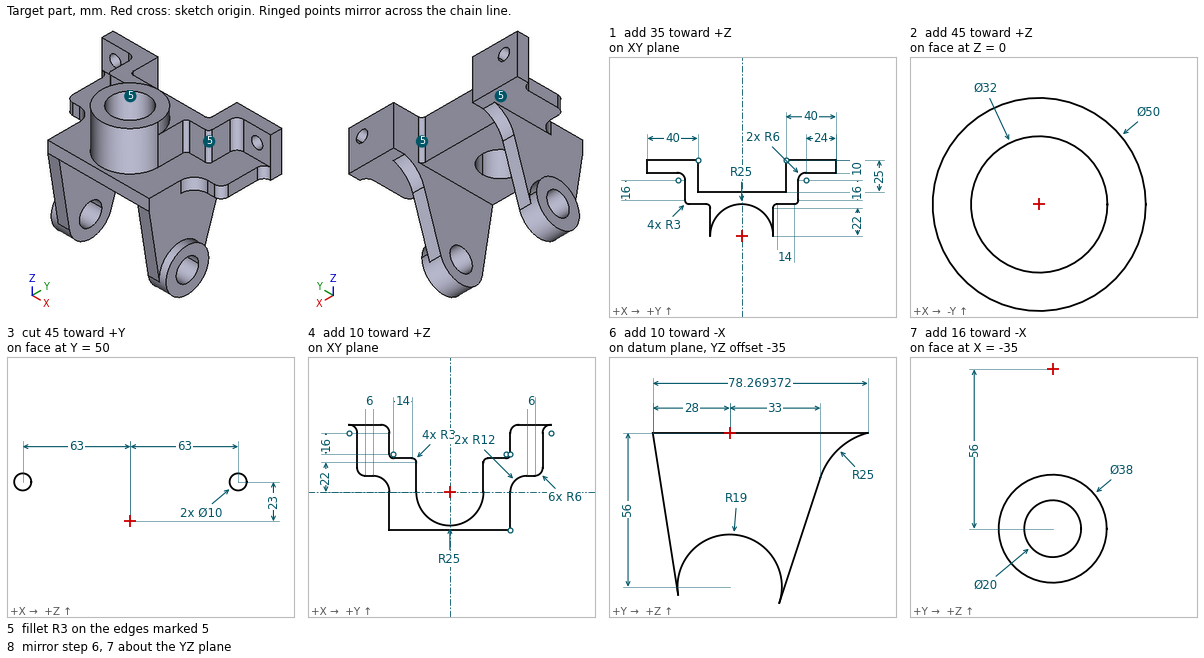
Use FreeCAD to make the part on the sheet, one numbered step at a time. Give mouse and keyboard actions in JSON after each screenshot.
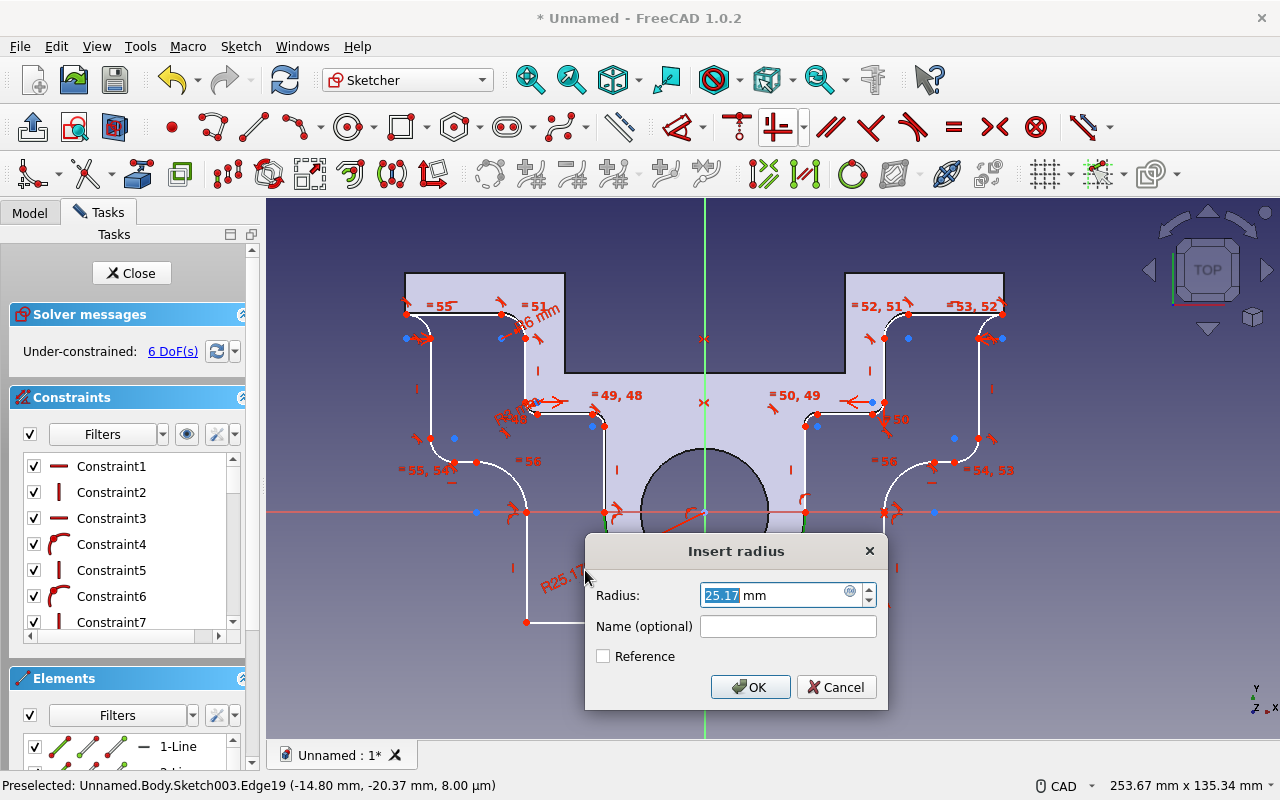
{"action": "type", "text": "25"}
{"action": "key", "text": "Return"}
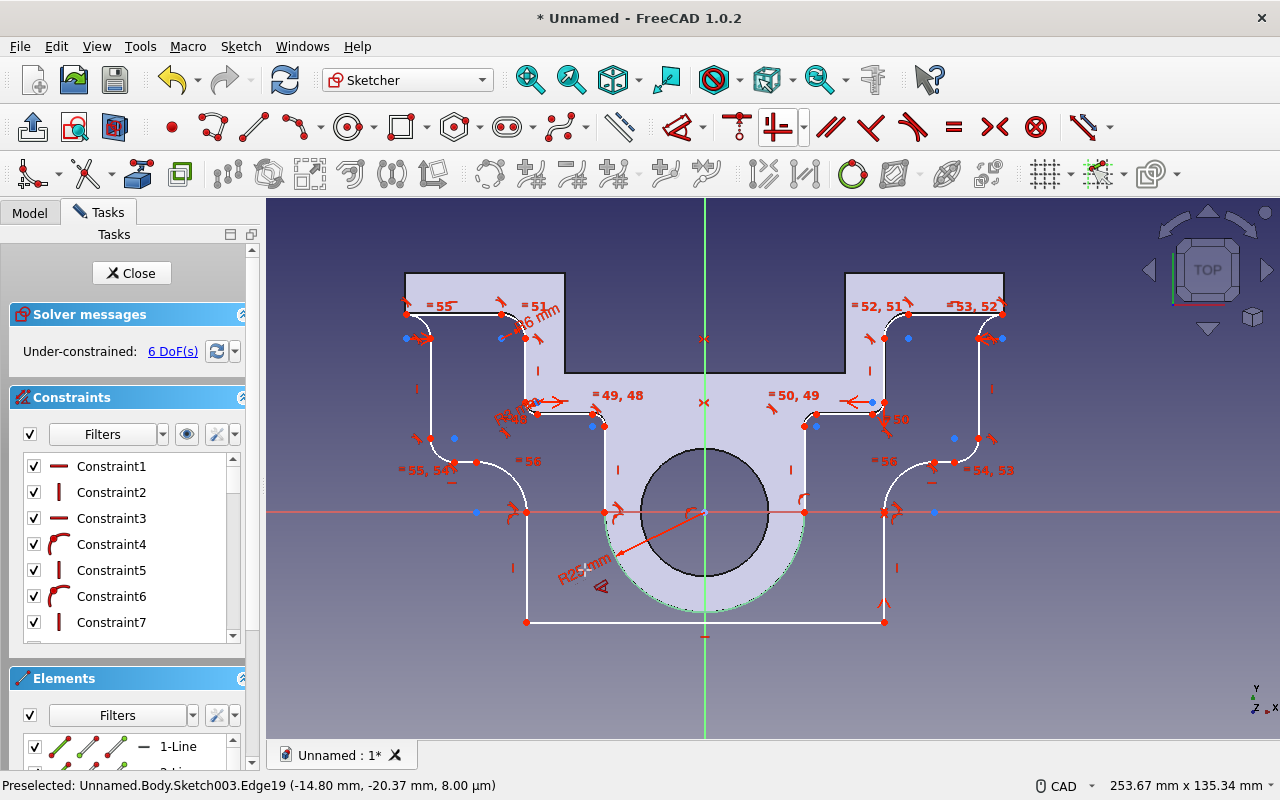
{"action": "left_click", "coordinate": [912, 468]}
{"action": "left_click", "coordinate": [898, 439]}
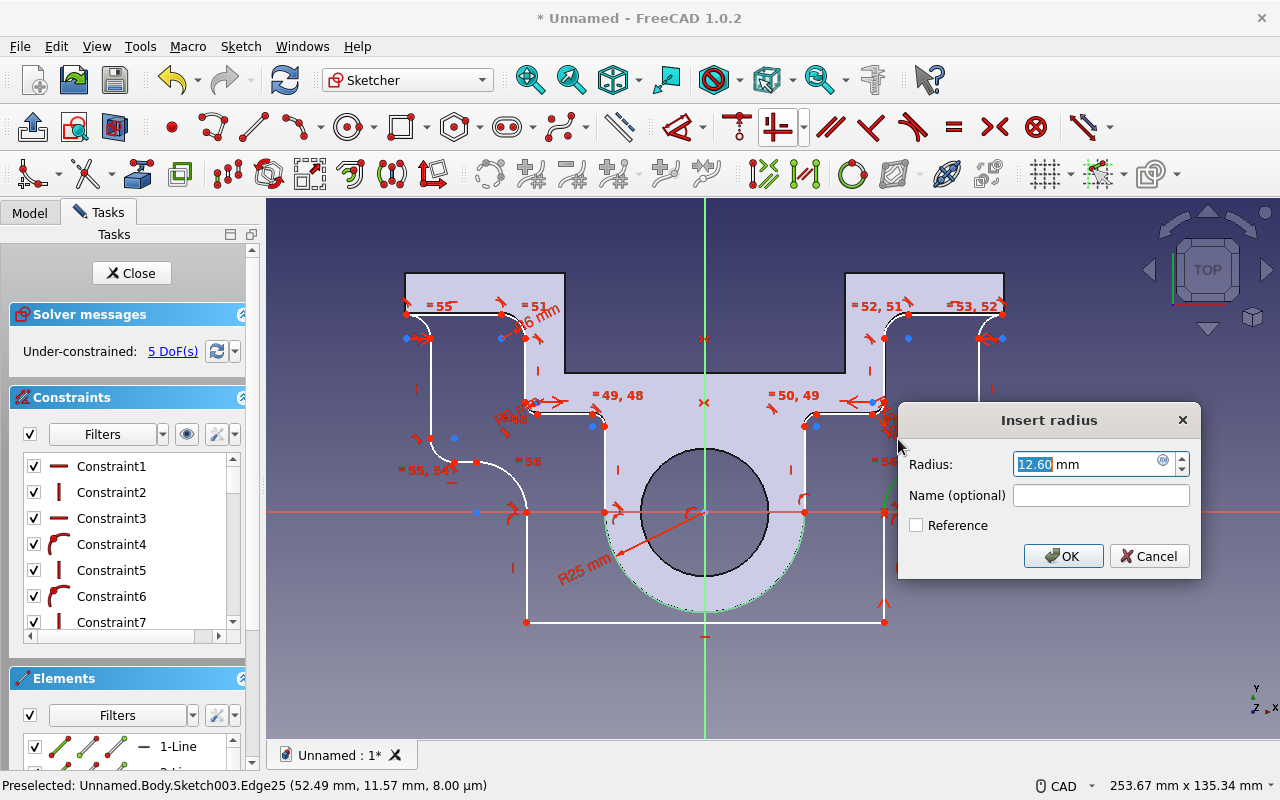
{"action": "type", "text": "12"}
{"action": "key", "text": "Return"}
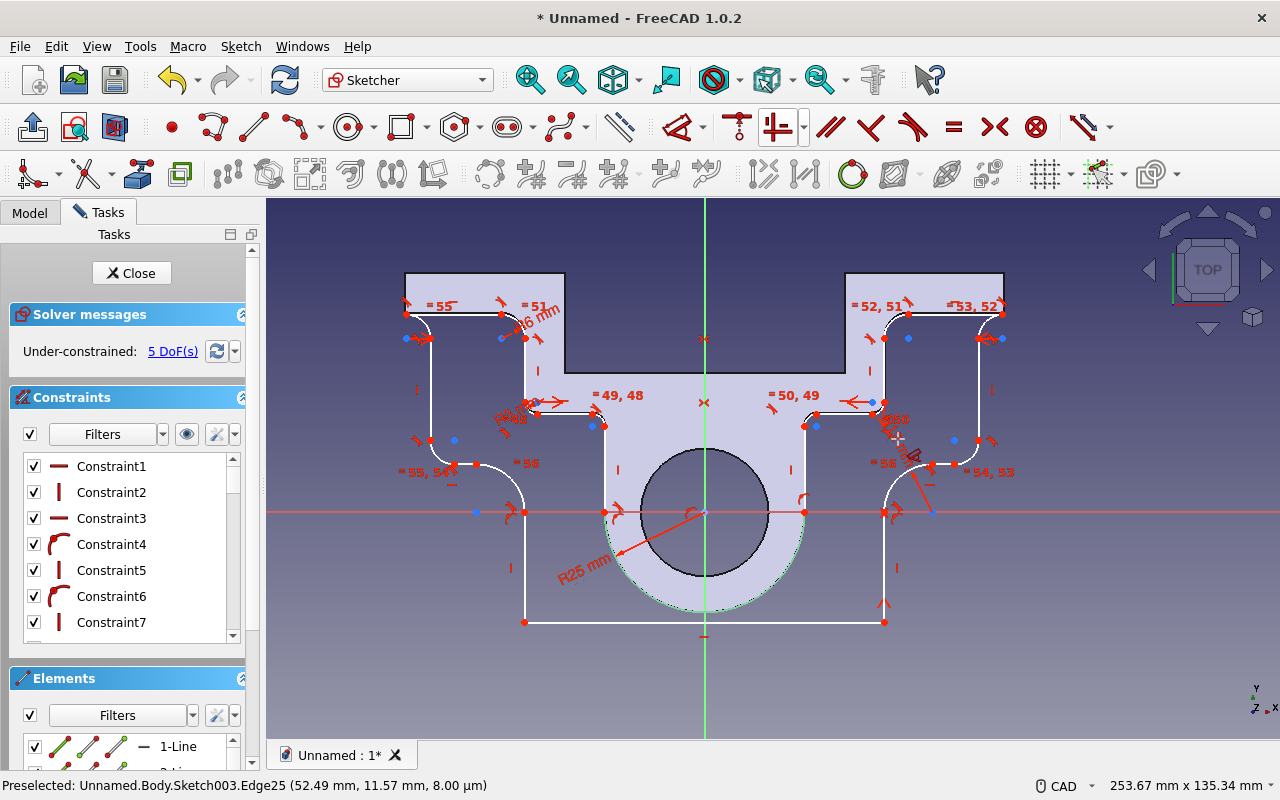
{"action": "scroll", "coordinate": [946, 464], "scroll_direction": "up", "scroll_amount": 3}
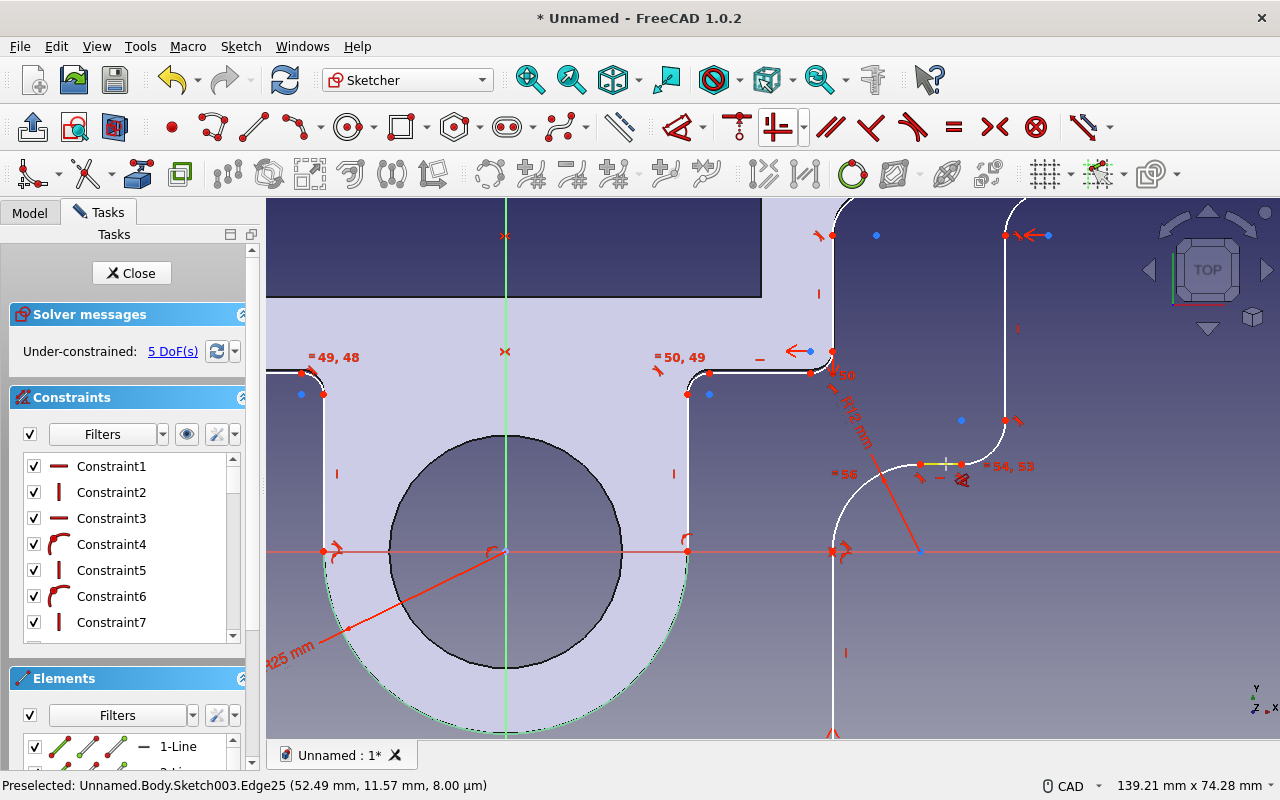
{"action": "left_click", "coordinate": [945, 464]}
{"action": "left_click", "coordinate": [941, 430]}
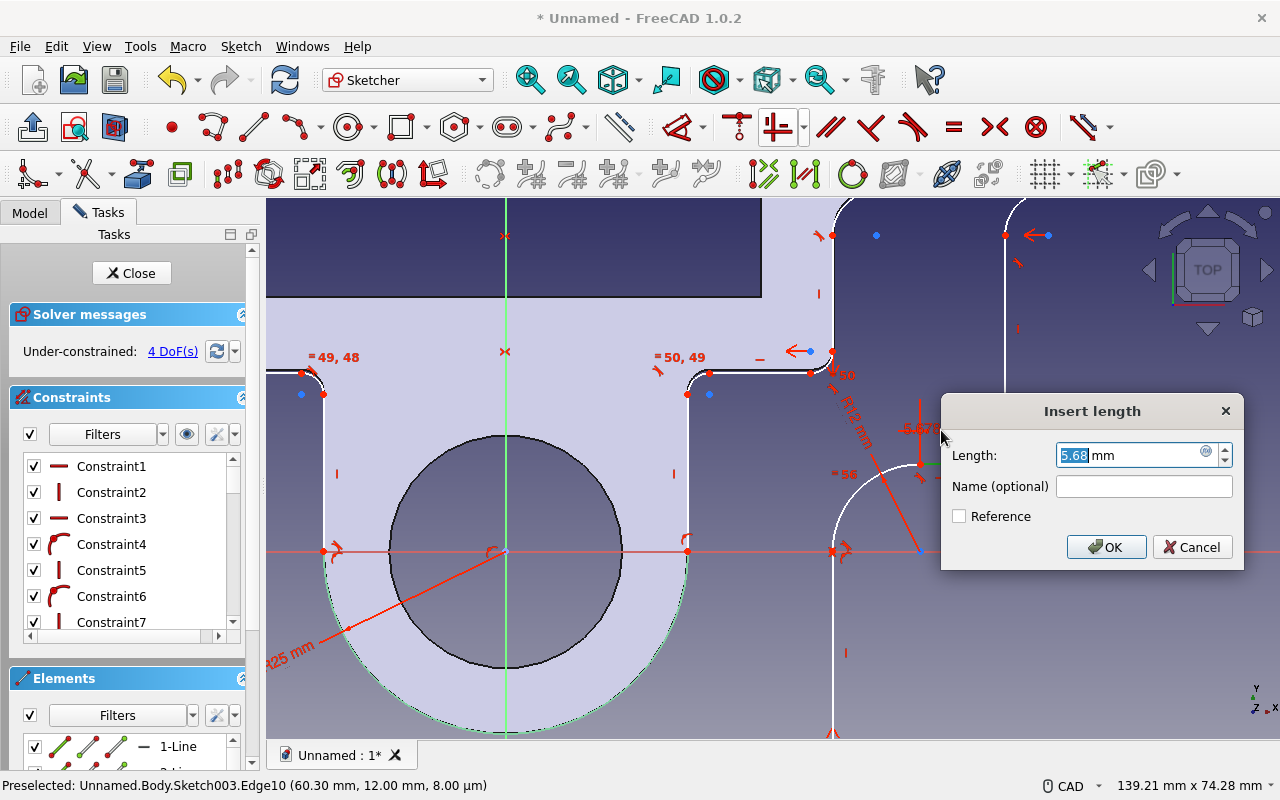
{"action": "type", "text": "6"}
{"action": "key", "text": "Return"}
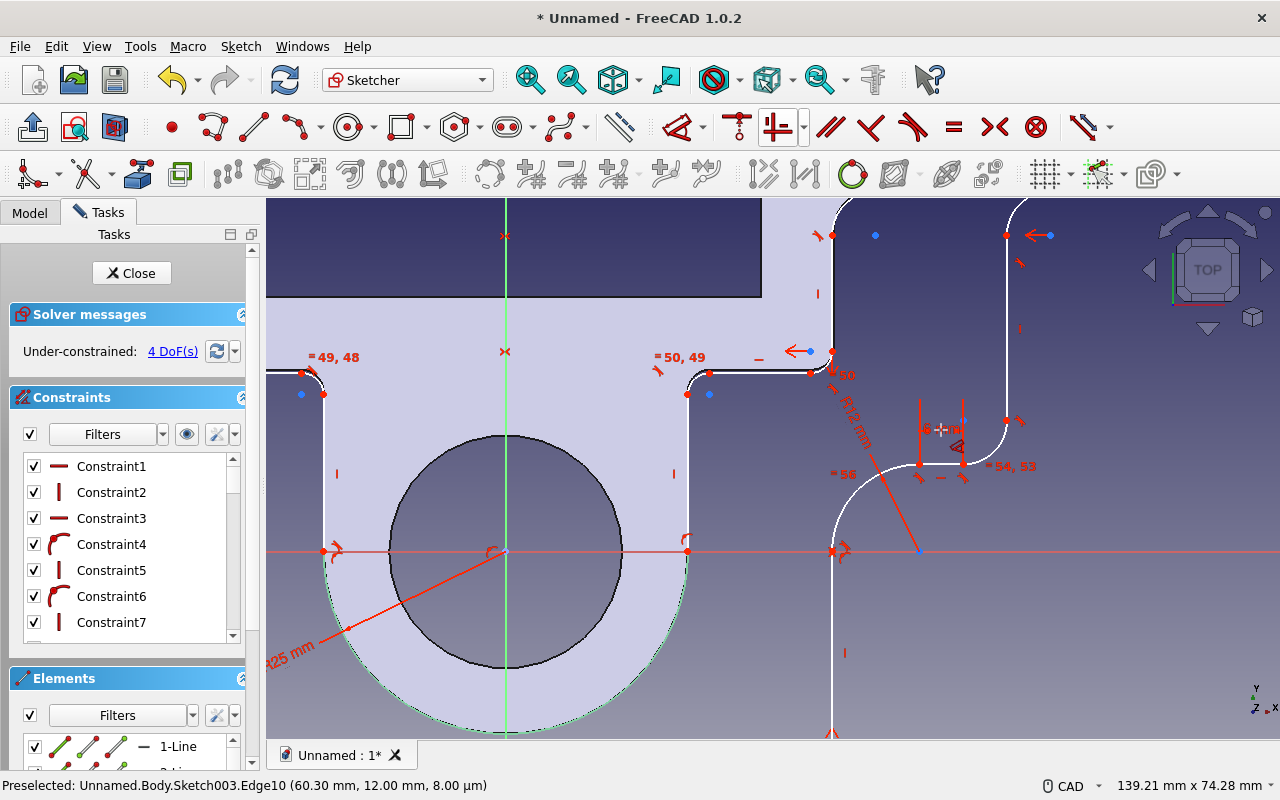
{"action": "scroll", "coordinate": [946, 465], "scroll_direction": "down", "scroll_amount": 3}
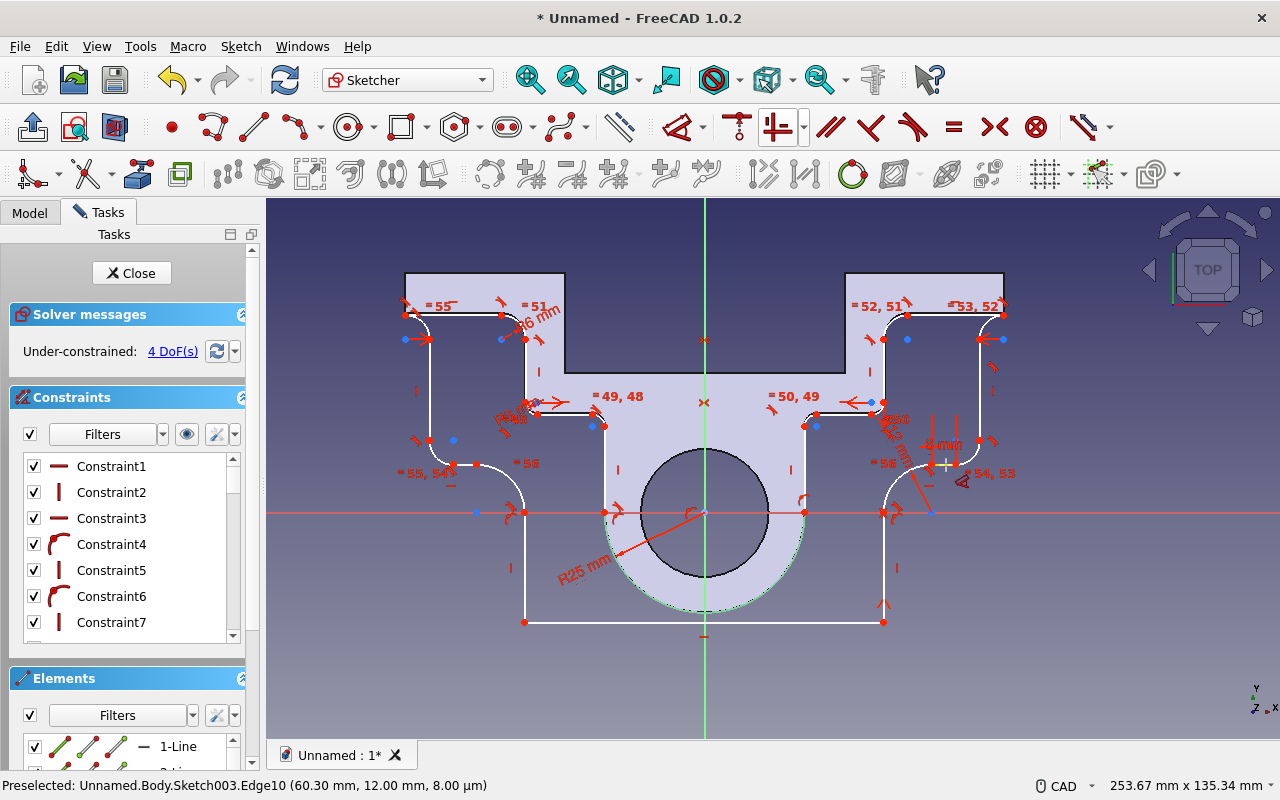
{"action": "scroll", "coordinate": [470, 465], "scroll_direction": "up", "scroll_amount": 4}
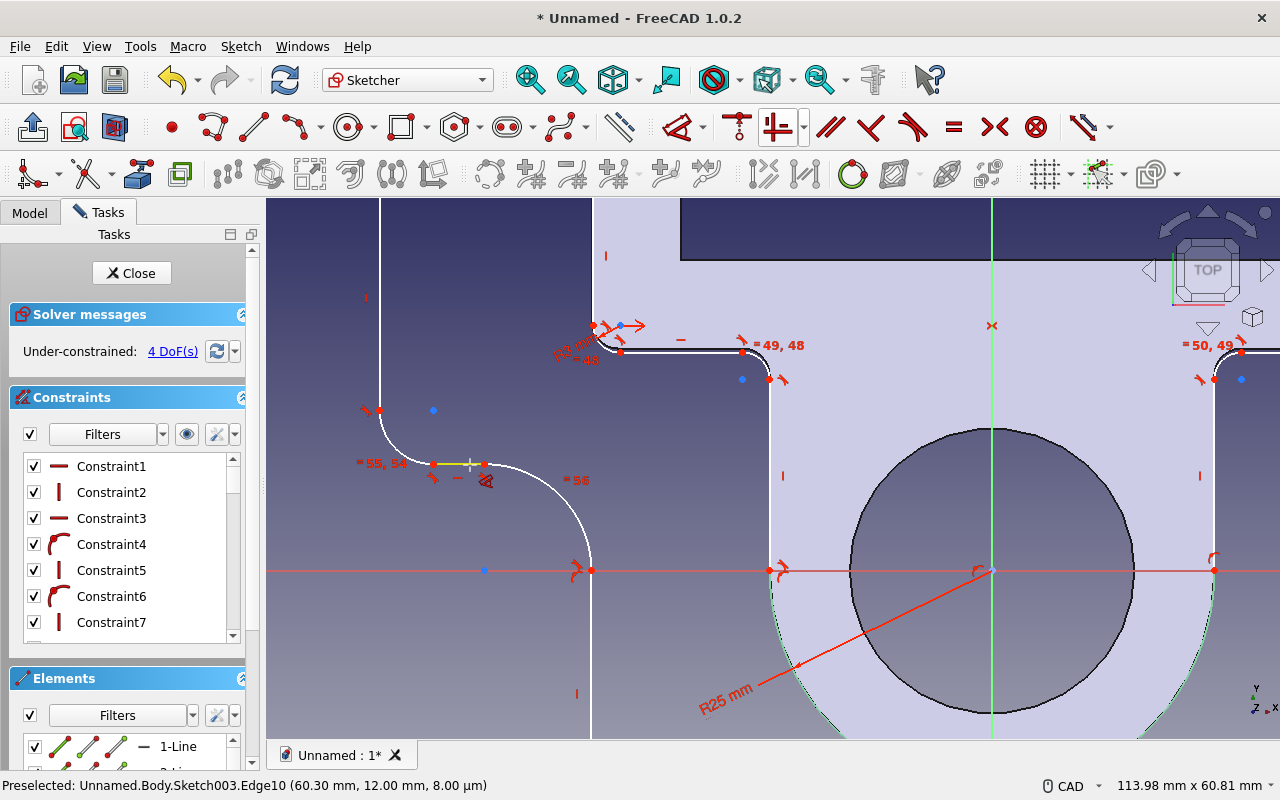
{"action": "left_click", "coordinate": [469, 464]}
{"action": "left_click", "coordinate": [459, 430]}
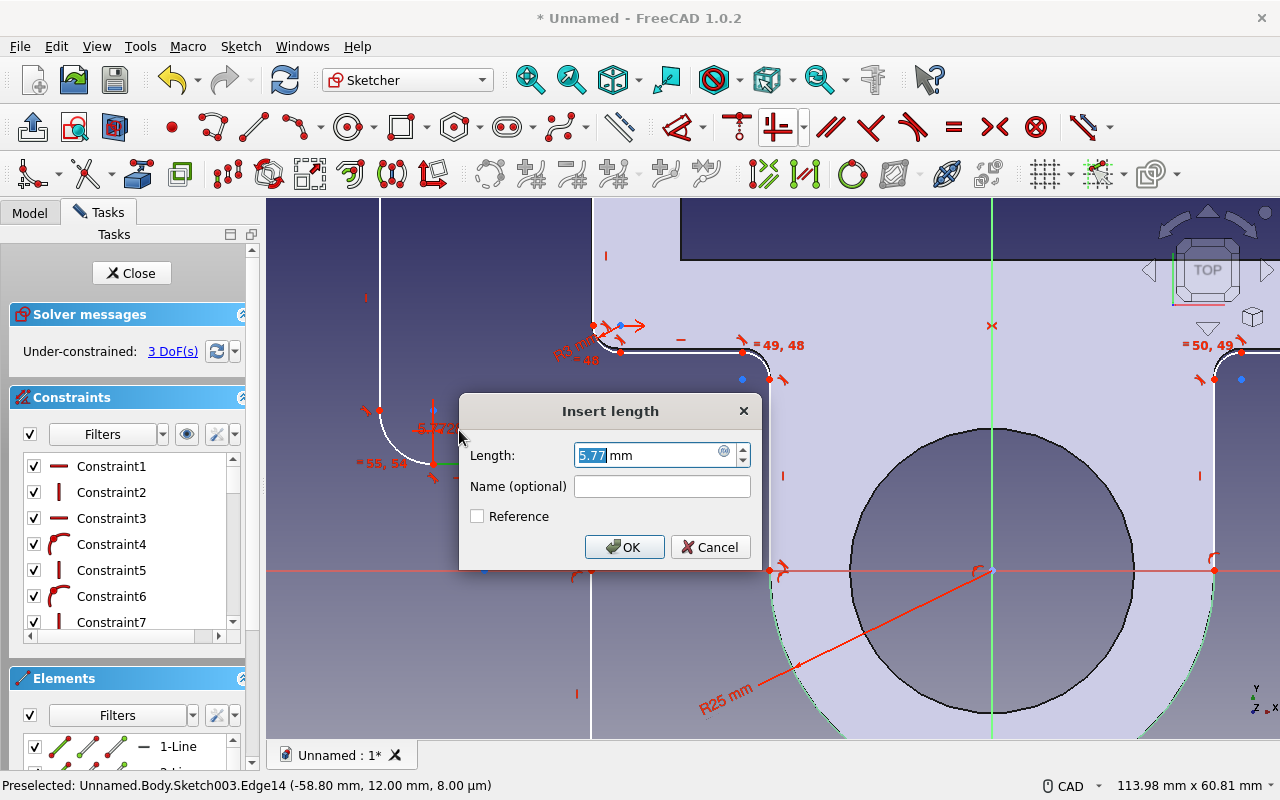
{"action": "type", "text": "6"}
{"action": "key", "text": "Return"}